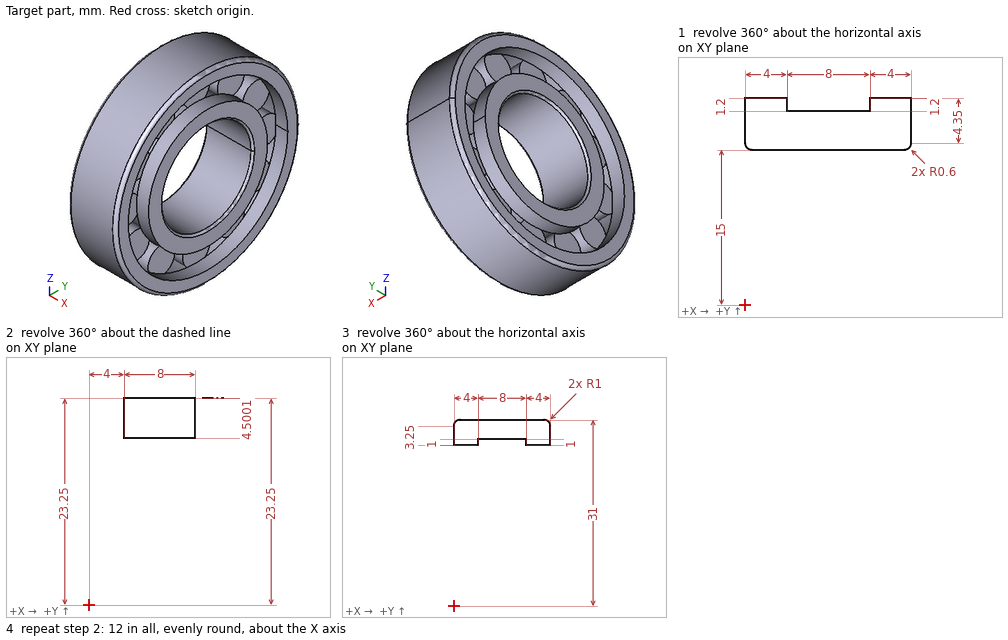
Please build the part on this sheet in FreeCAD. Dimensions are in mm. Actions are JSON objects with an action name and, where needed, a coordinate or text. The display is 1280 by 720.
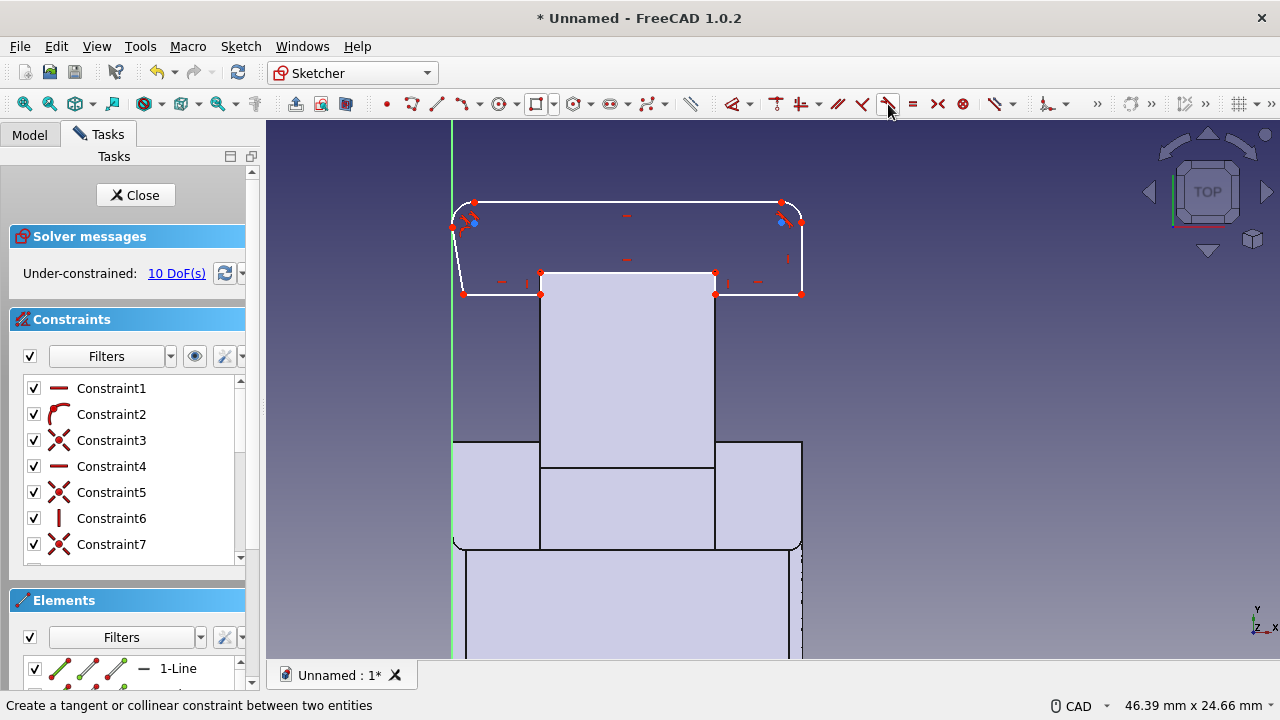
{"action": "left_click", "coordinate": [456, 248]}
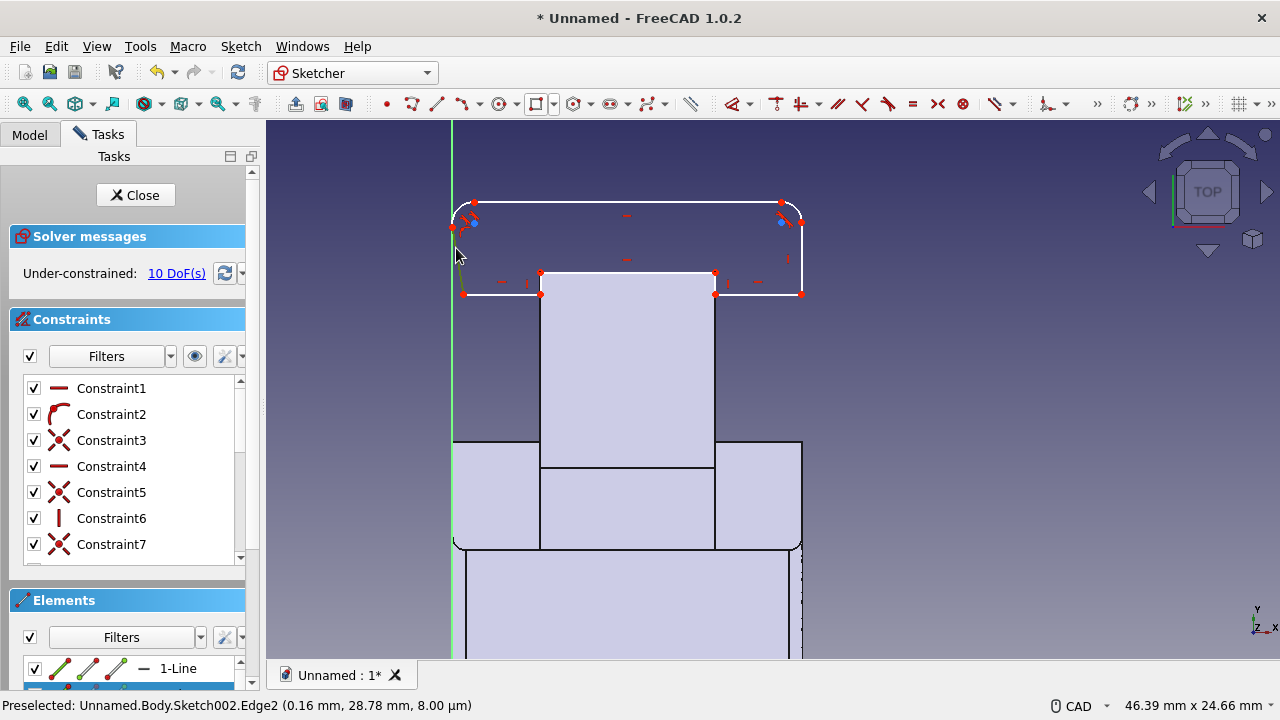
{"action": "left_click", "coordinate": [818, 104]}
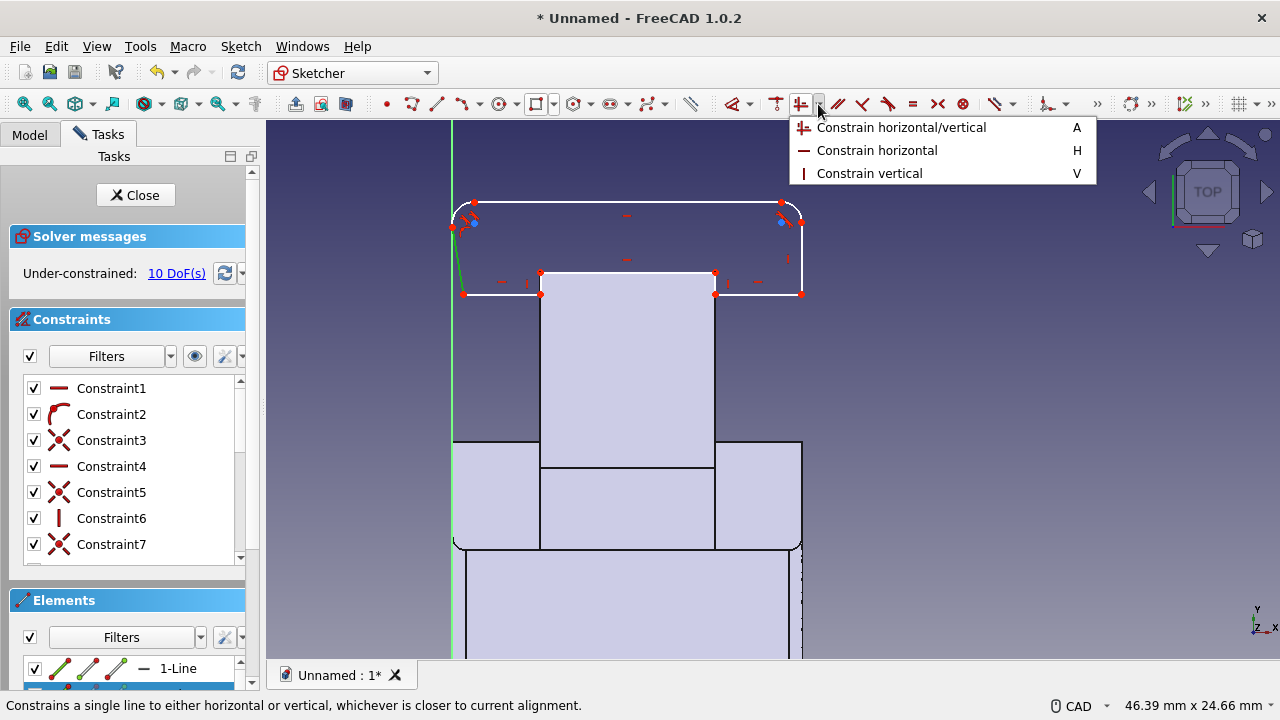
{"action": "left_click", "coordinate": [943, 174]}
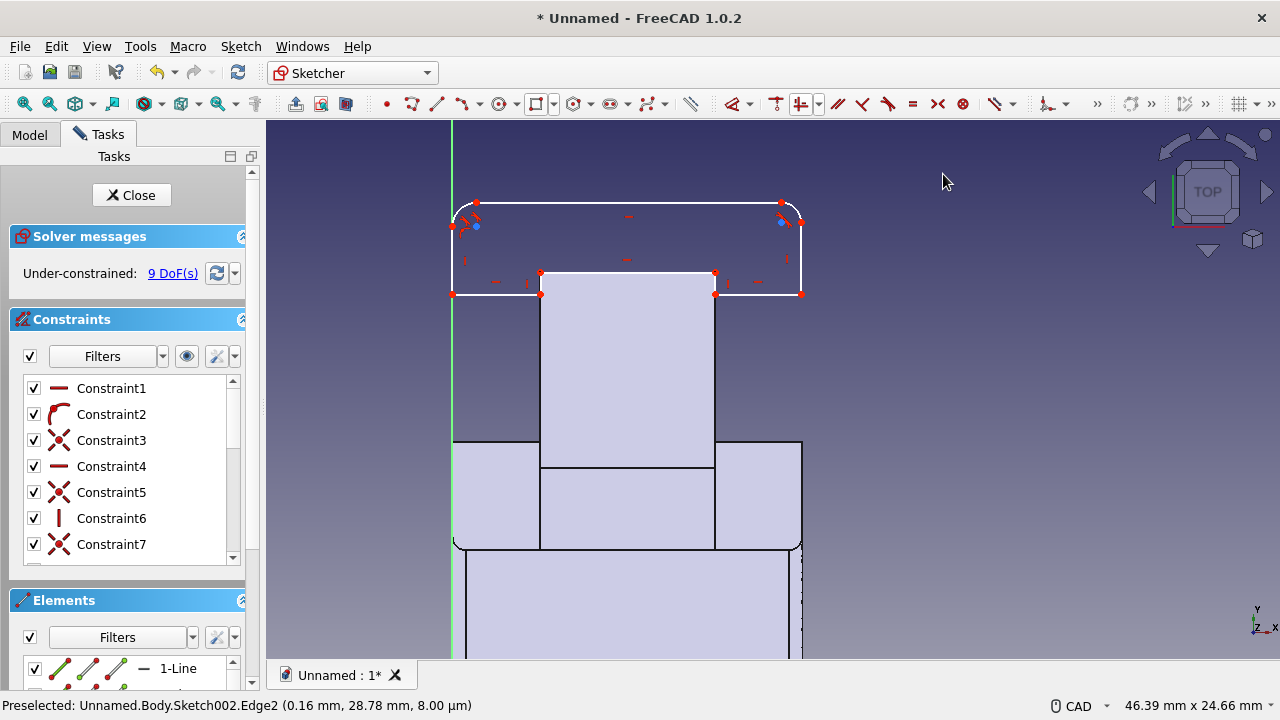
{"action": "scroll", "coordinate": [466, 205], "scroll_direction": "up", "scroll_amount": 2}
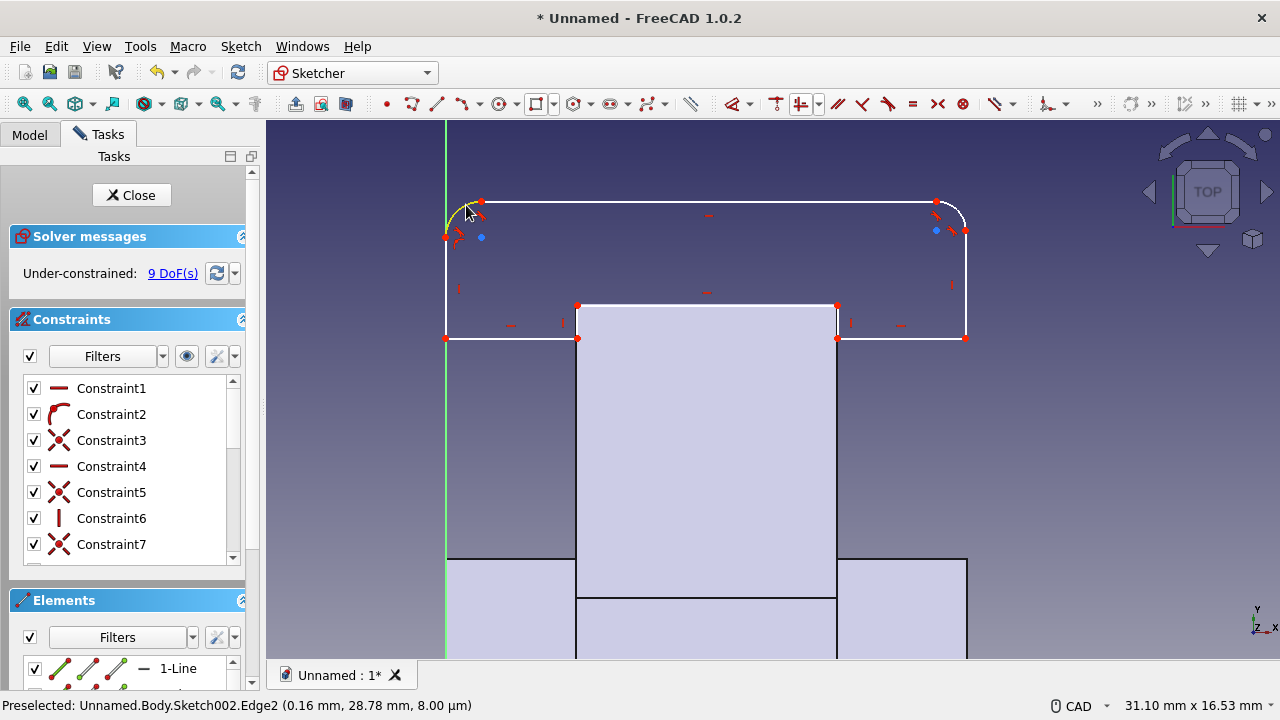
{"action": "left_click", "coordinate": [465, 206]}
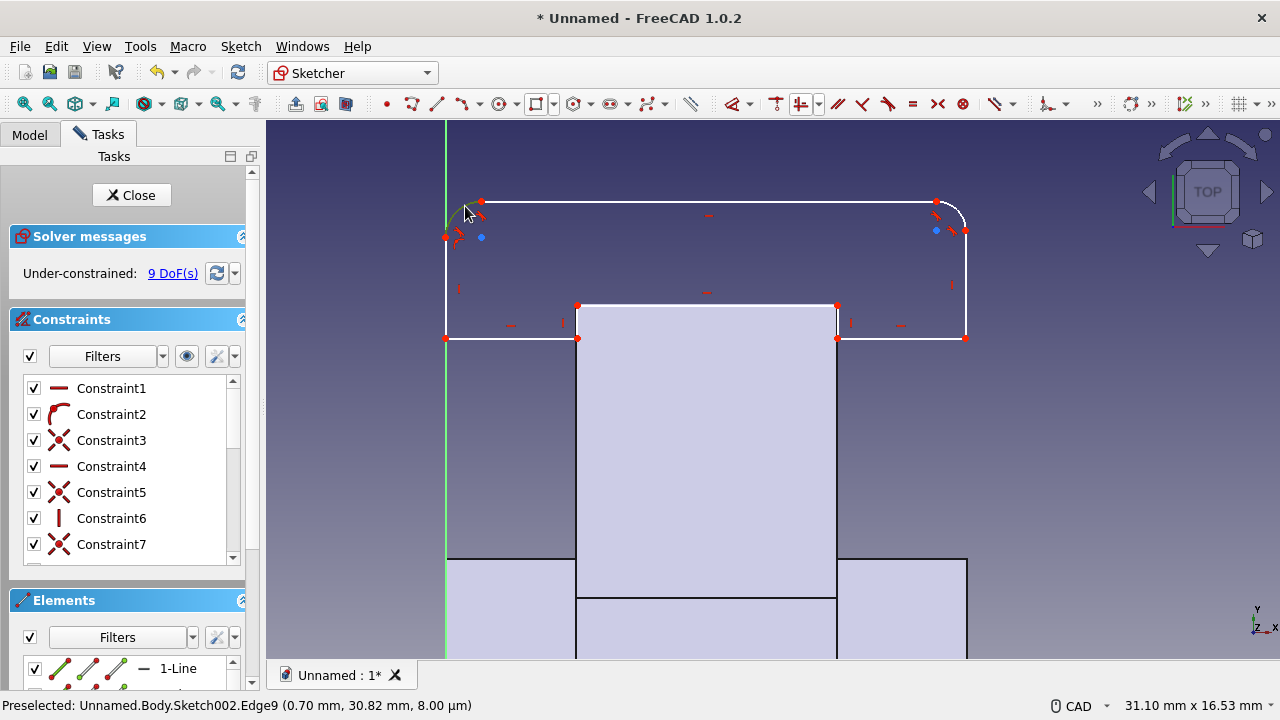
{"action": "left_click", "coordinate": [963, 217]}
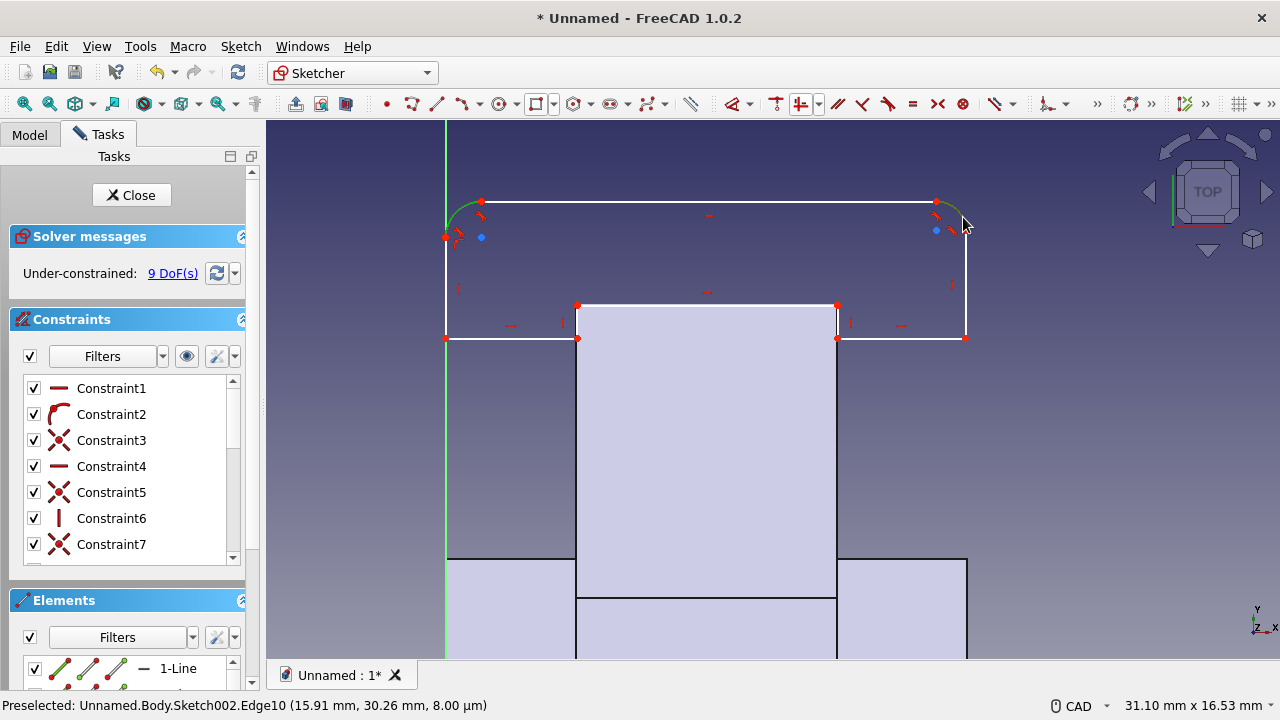
{"action": "left_click", "coordinate": [913, 104]}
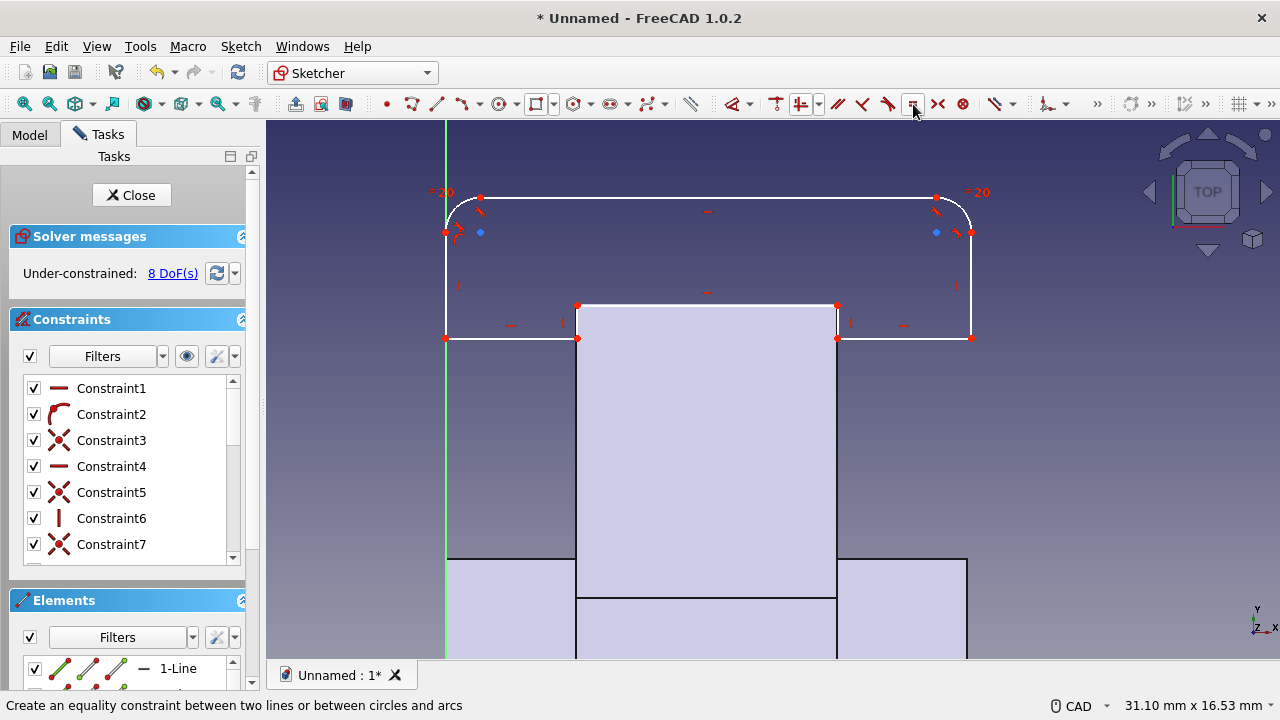
{"action": "left_click", "coordinate": [732, 104]}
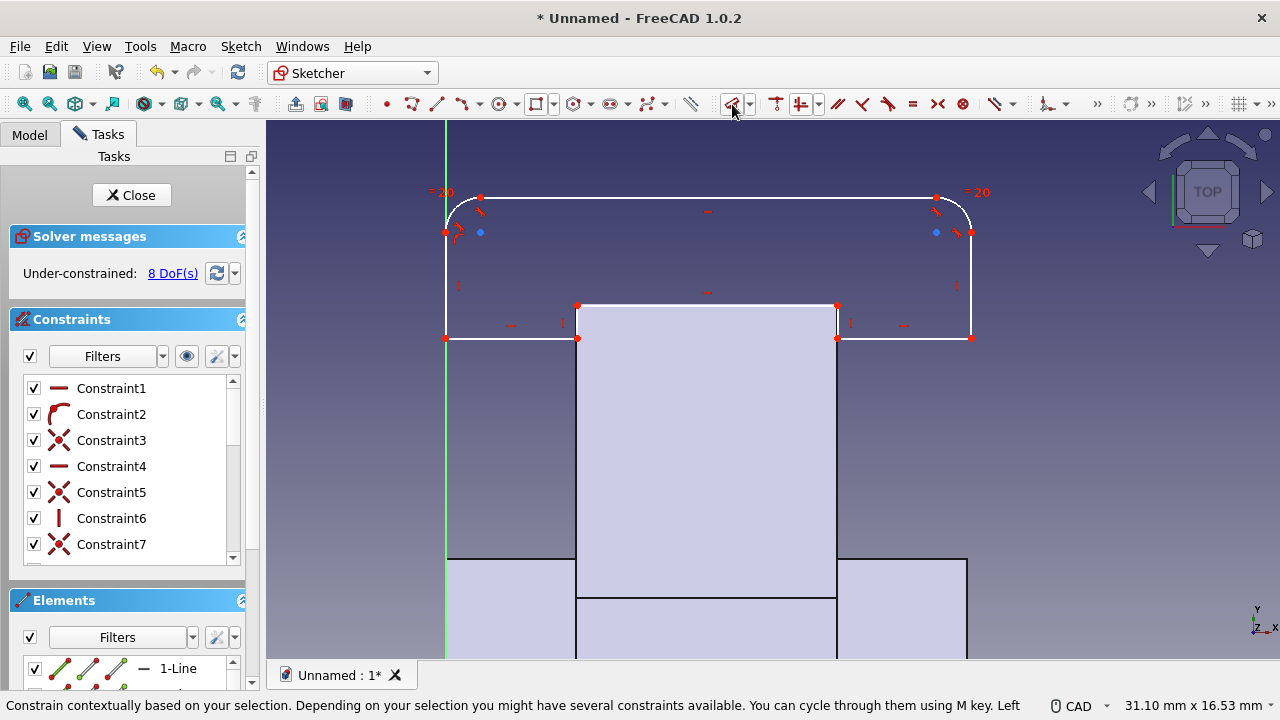
{"action": "left_click", "coordinate": [465, 202]}
{"action": "left_click", "coordinate": [483, 166]}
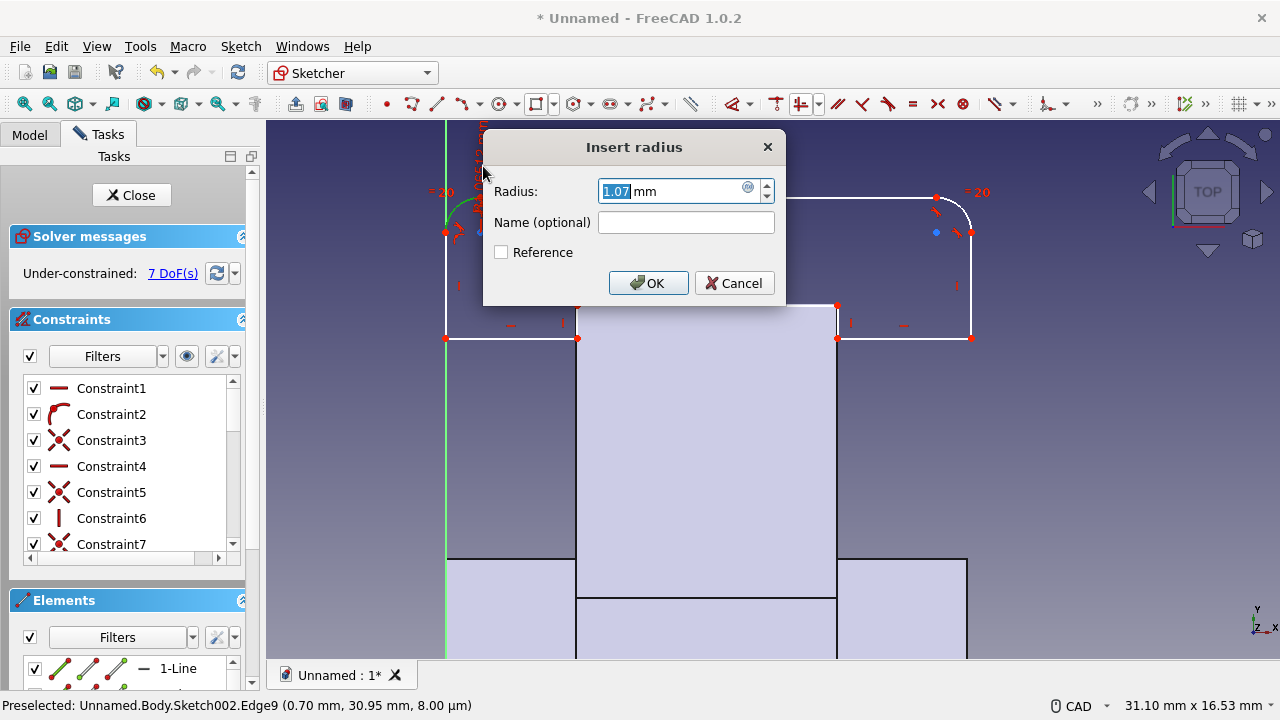
{"action": "type", "text": "1"}
{"action": "key", "text": "Return"}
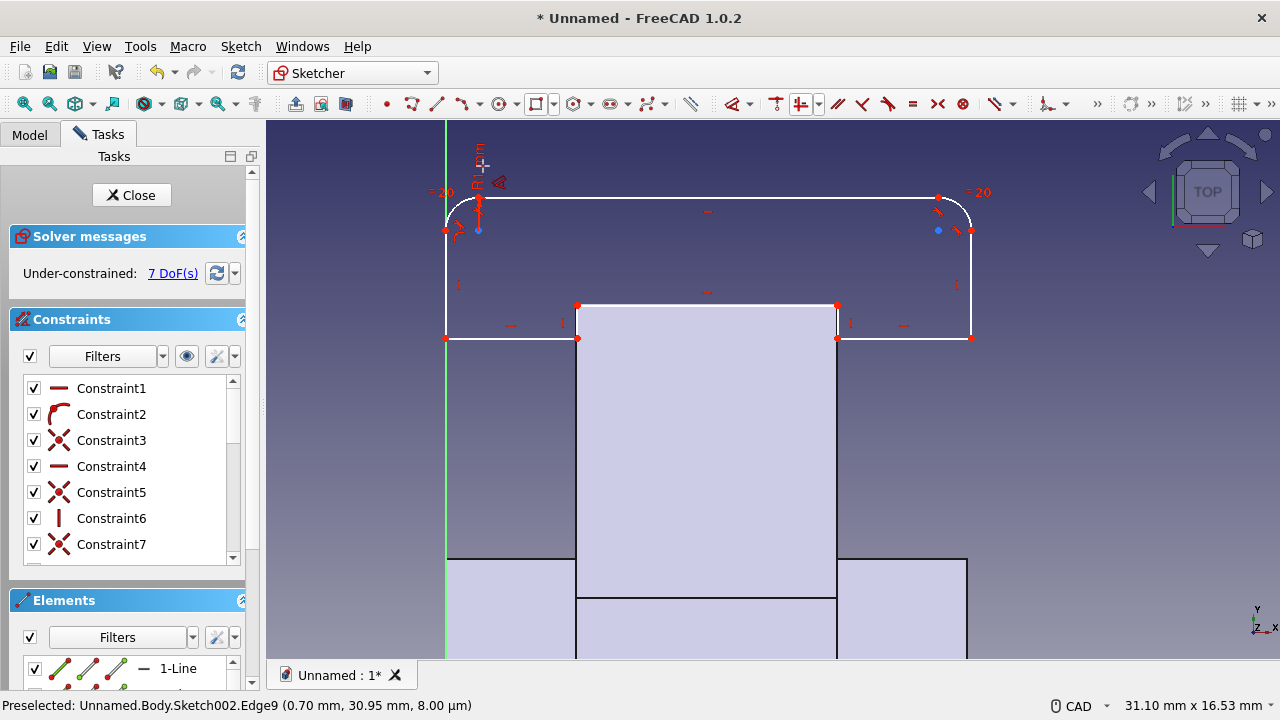
{"action": "left_click", "coordinate": [485, 339]}
{"action": "left_click", "coordinate": [511, 305]}